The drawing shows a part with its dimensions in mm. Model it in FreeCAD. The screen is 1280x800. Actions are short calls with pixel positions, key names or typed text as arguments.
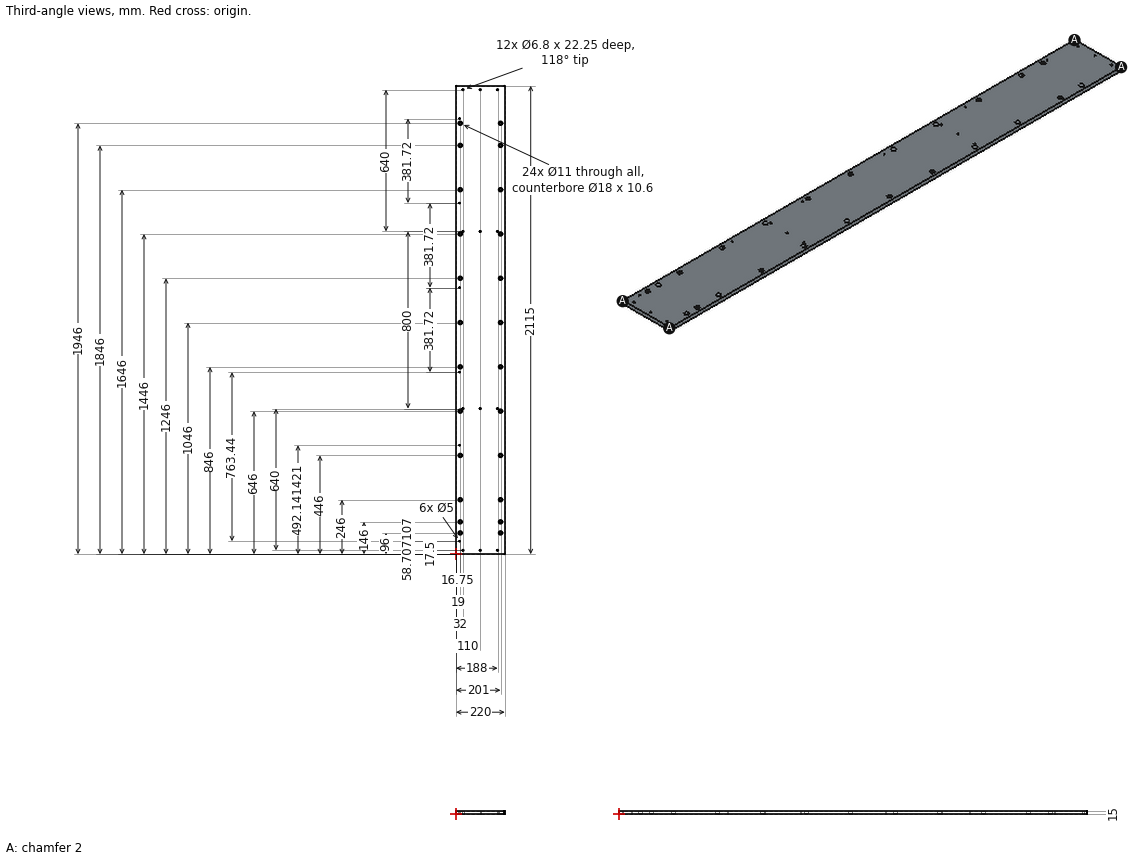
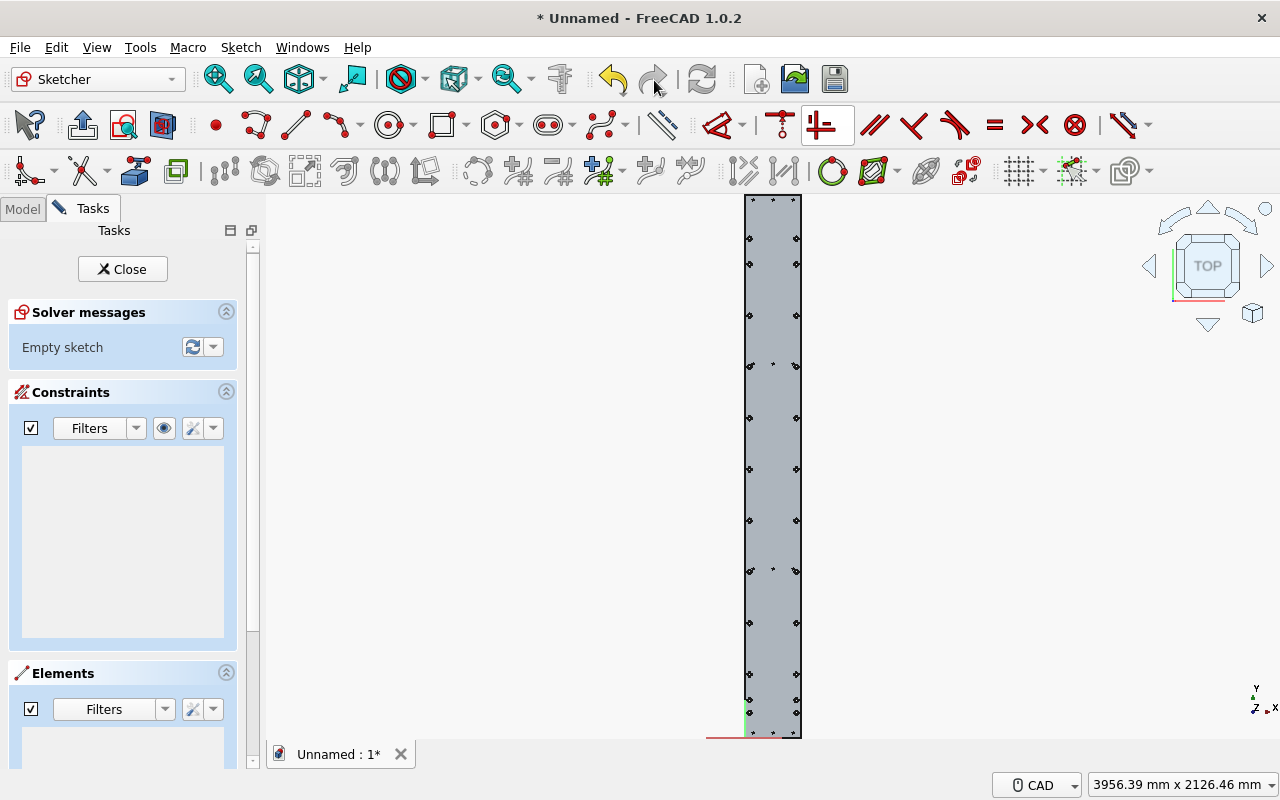
scroll(618, 429, down, 2)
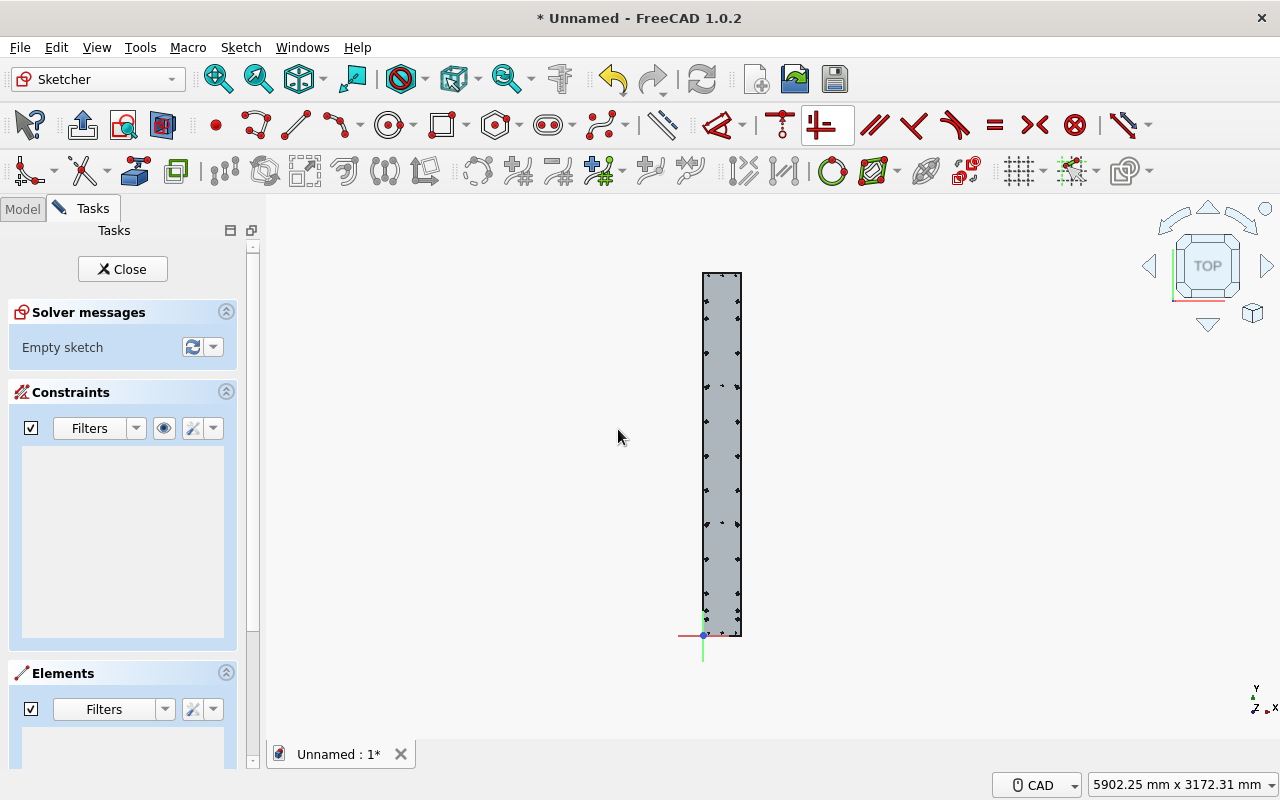
click(390, 126)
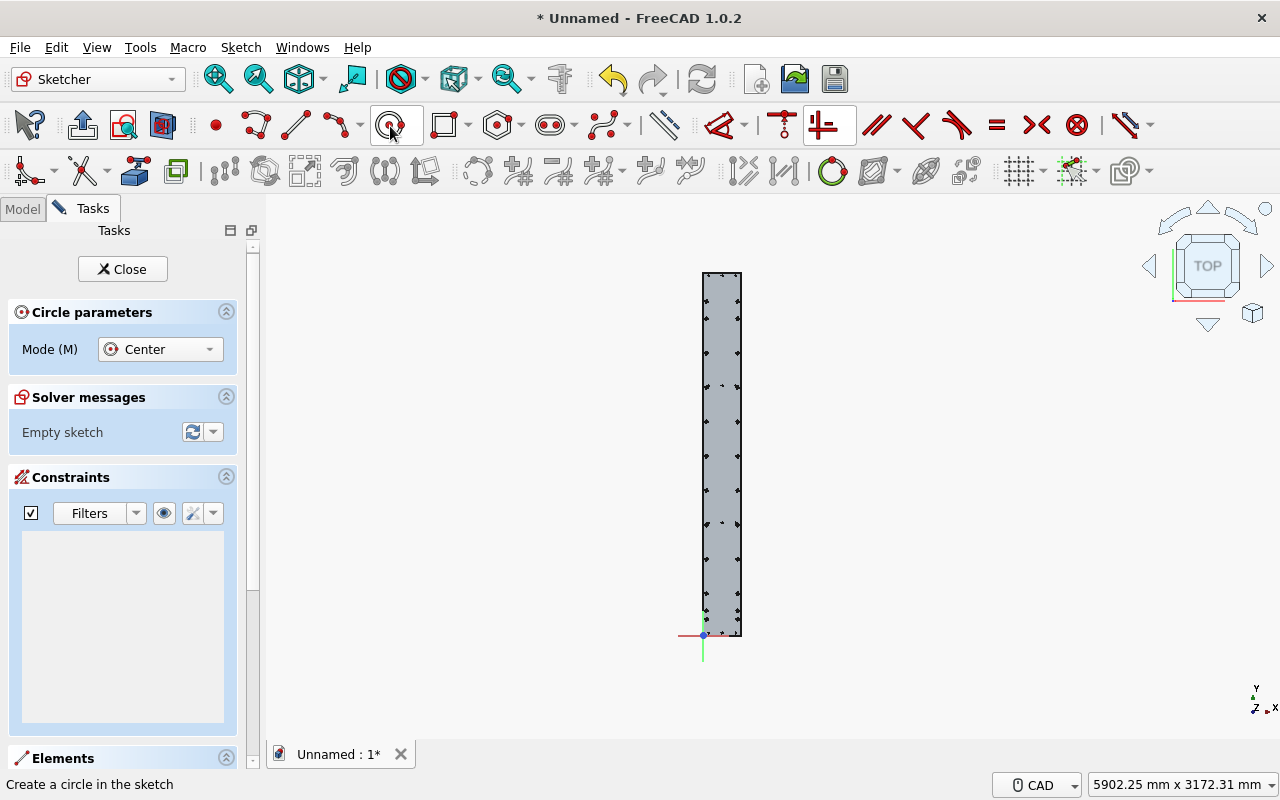
scroll(706, 626, up, 20)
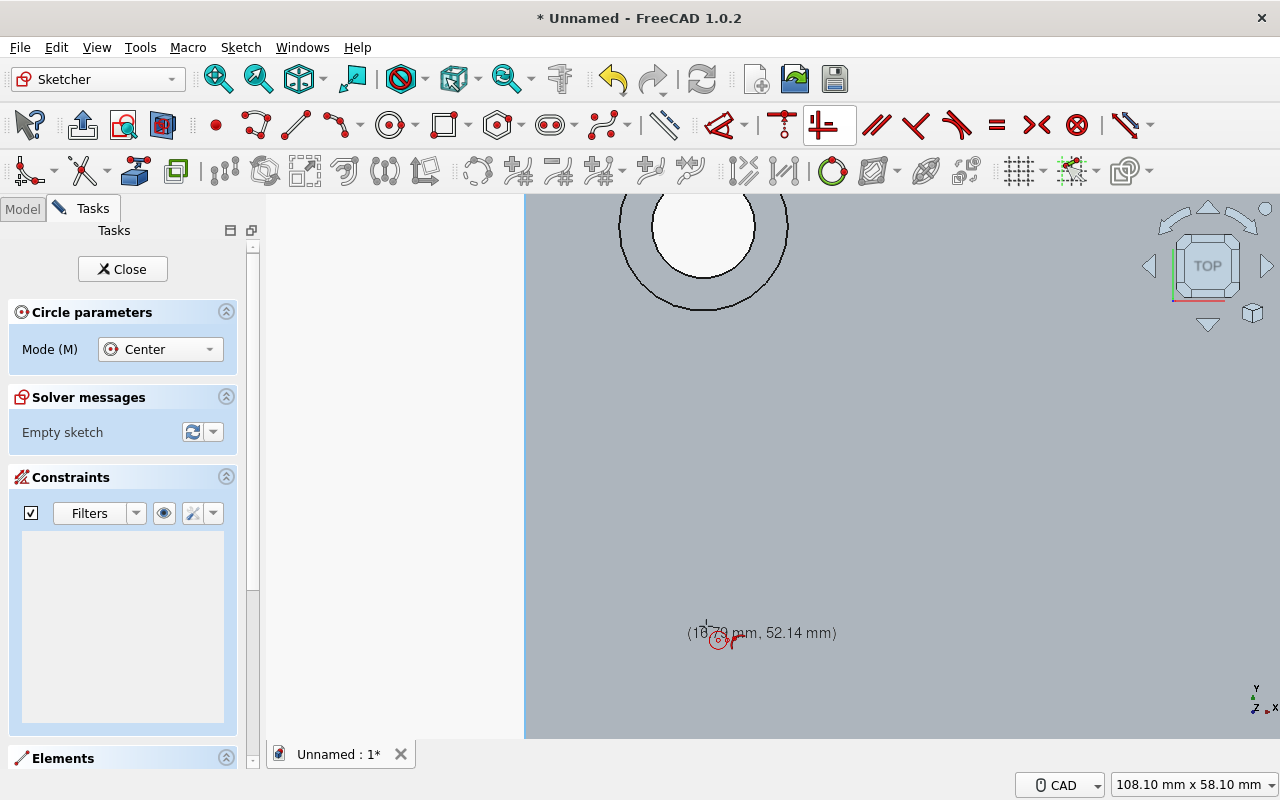
scroll(704, 466, down, 15)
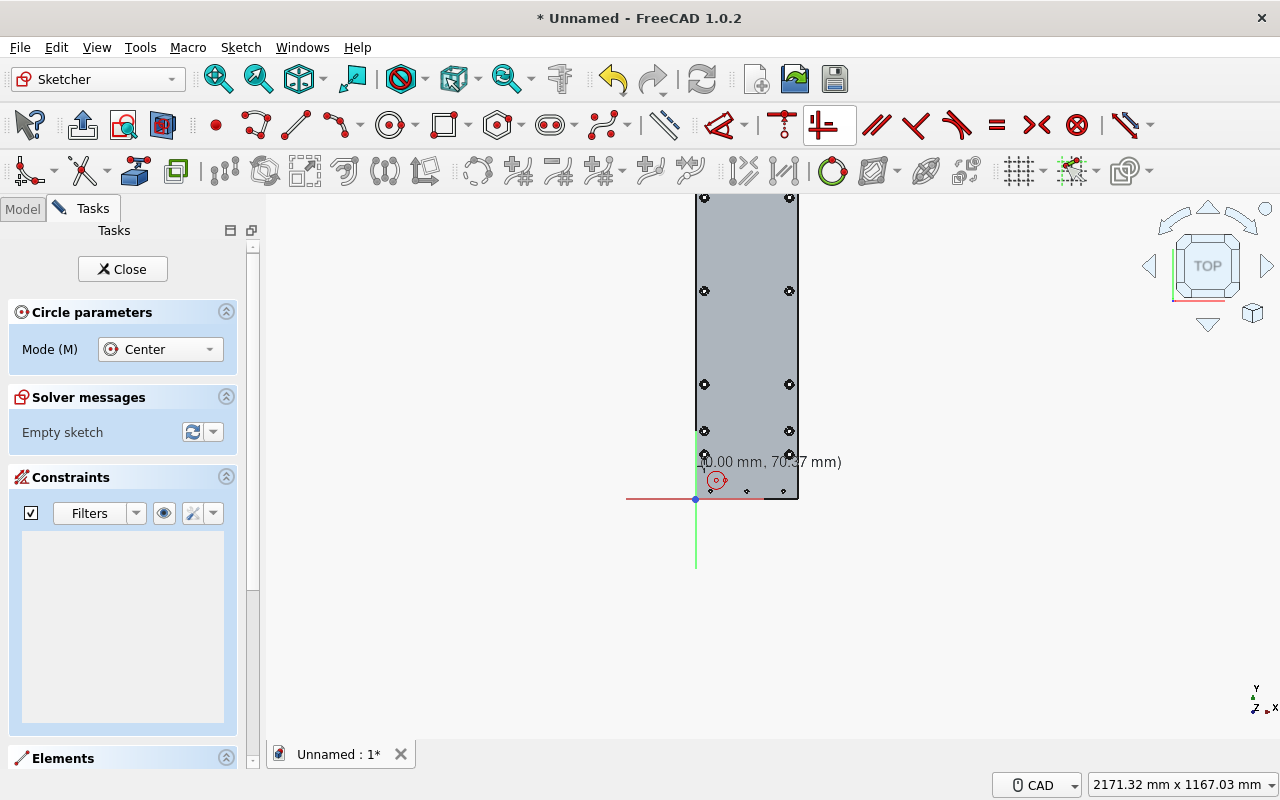
scroll(707, 711, down, 5)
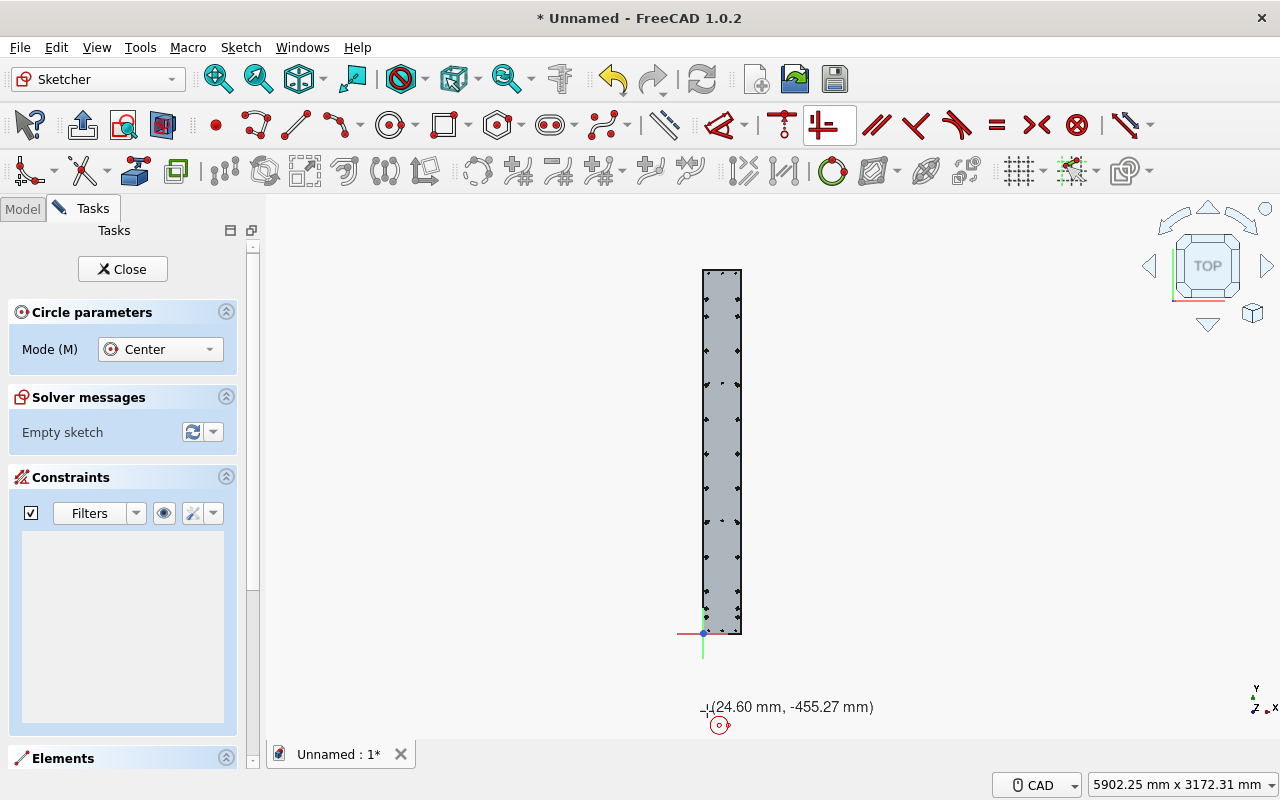
scroll(706, 624, up, 9)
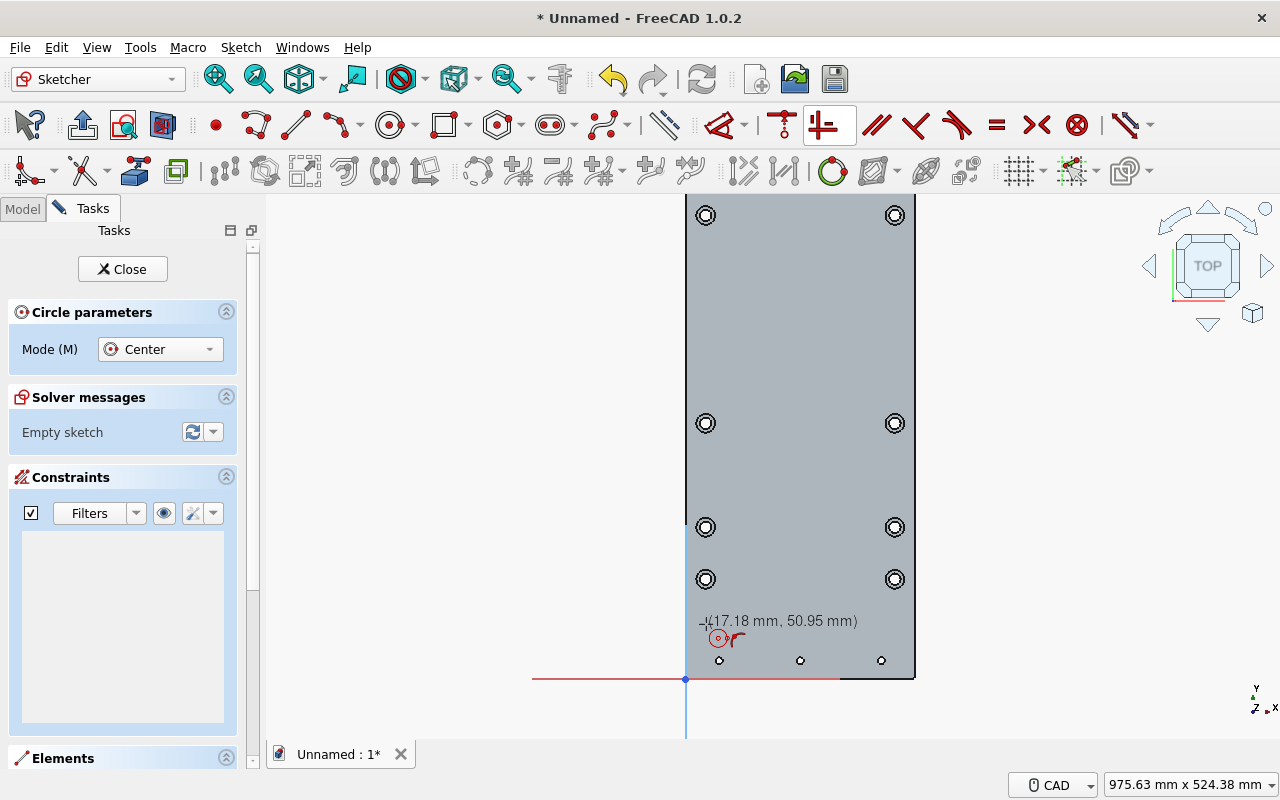
click(703, 618)
move(705, 616)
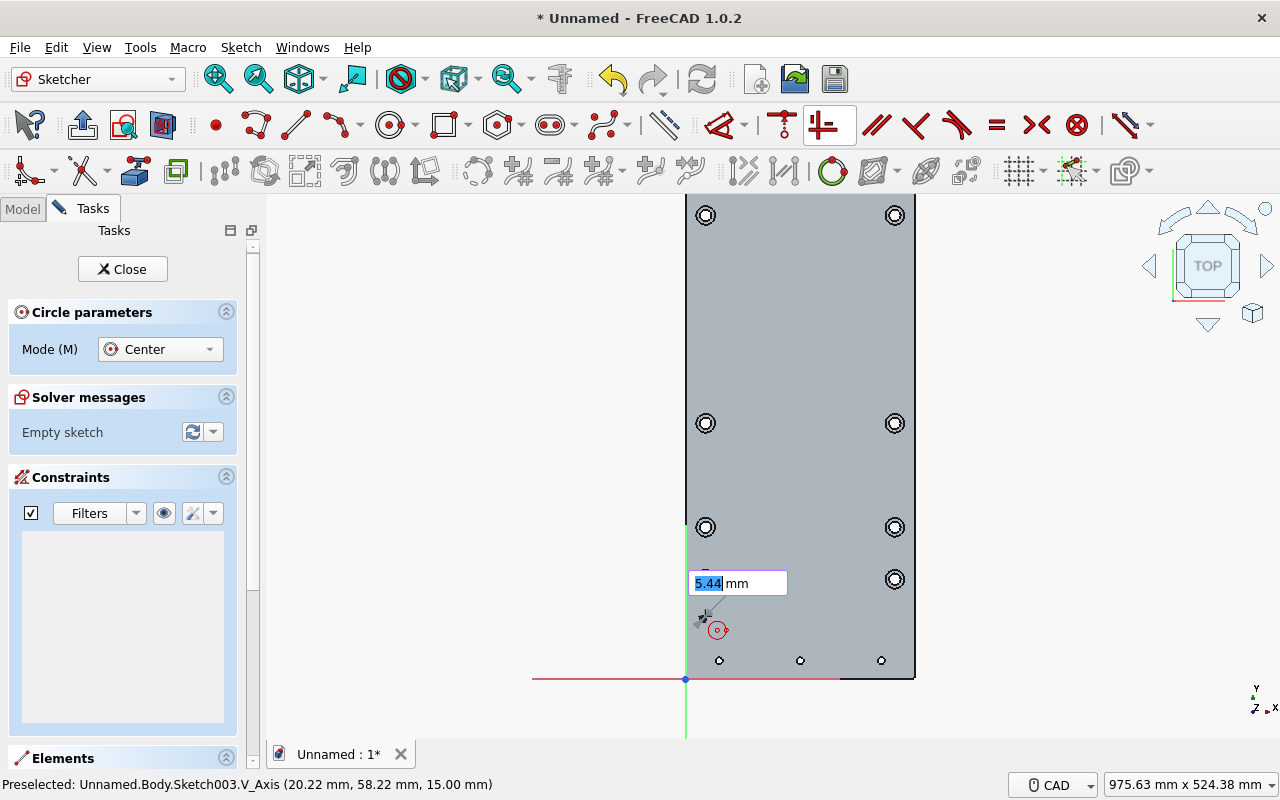
text(5)
key(Return)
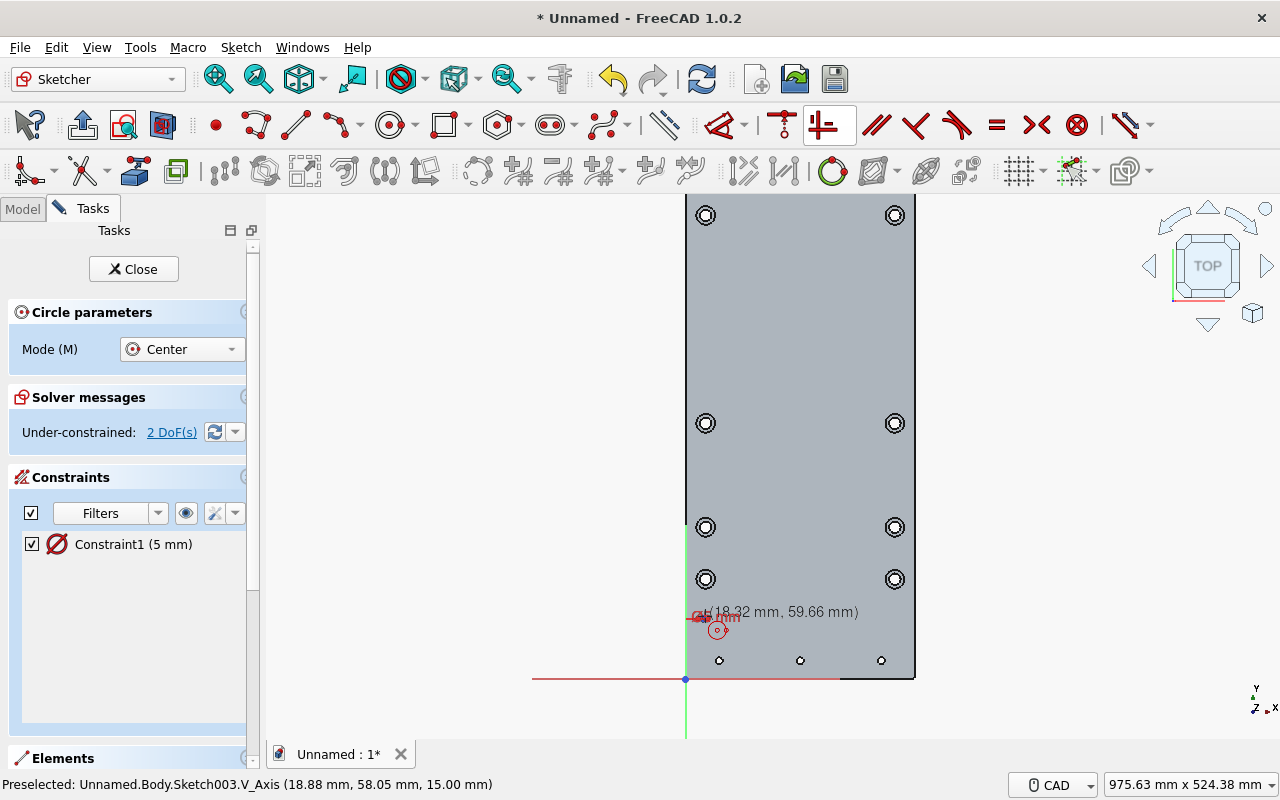
scroll(706, 627, down, 9)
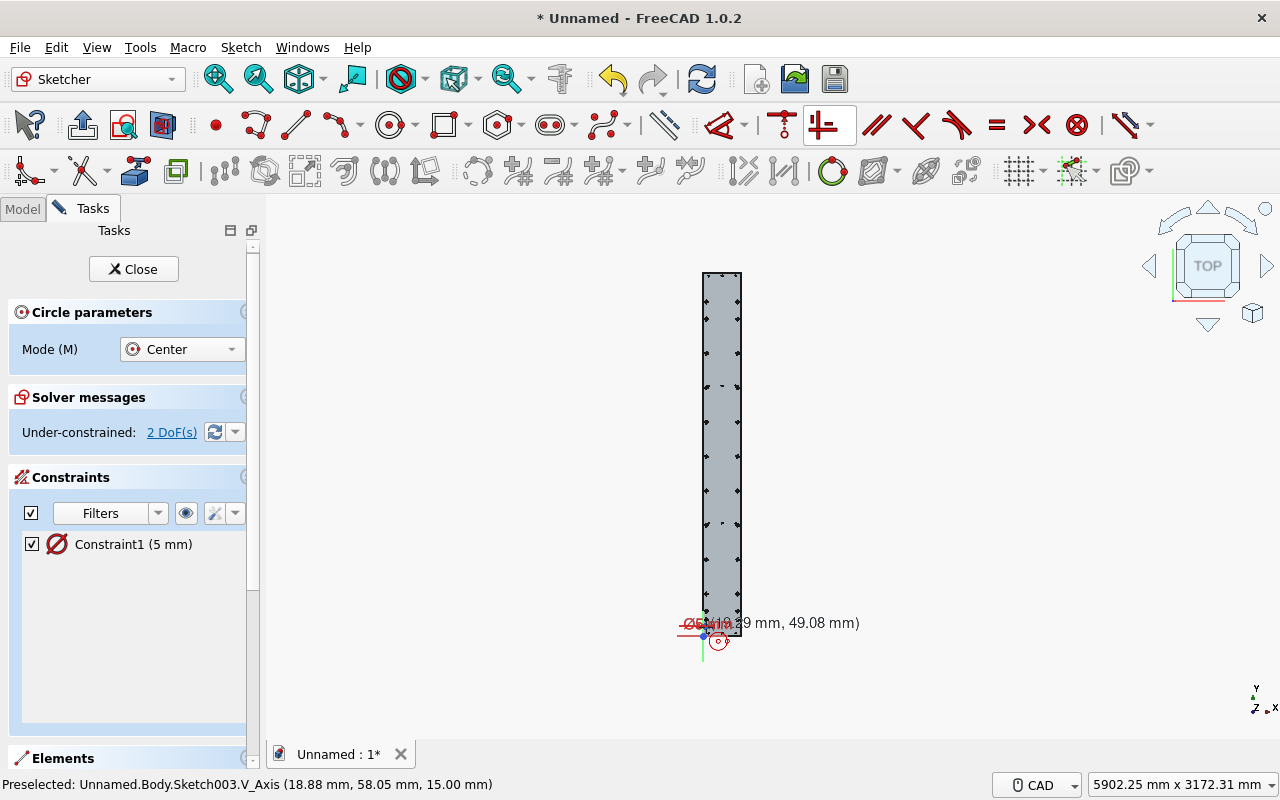
scroll(706, 552, up, 20)